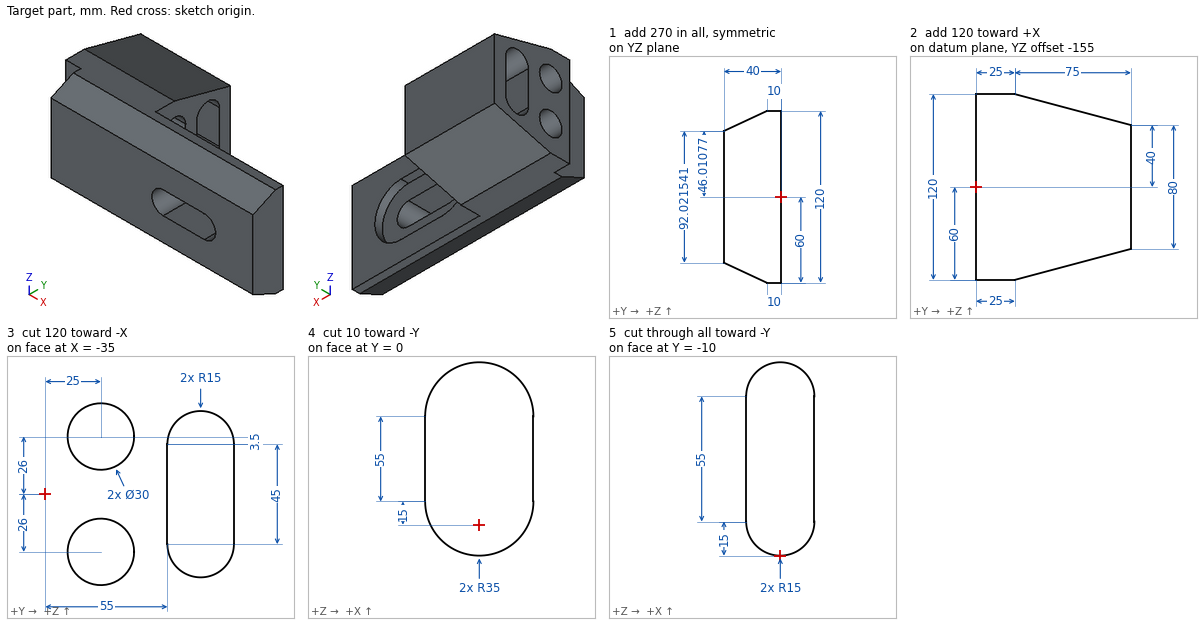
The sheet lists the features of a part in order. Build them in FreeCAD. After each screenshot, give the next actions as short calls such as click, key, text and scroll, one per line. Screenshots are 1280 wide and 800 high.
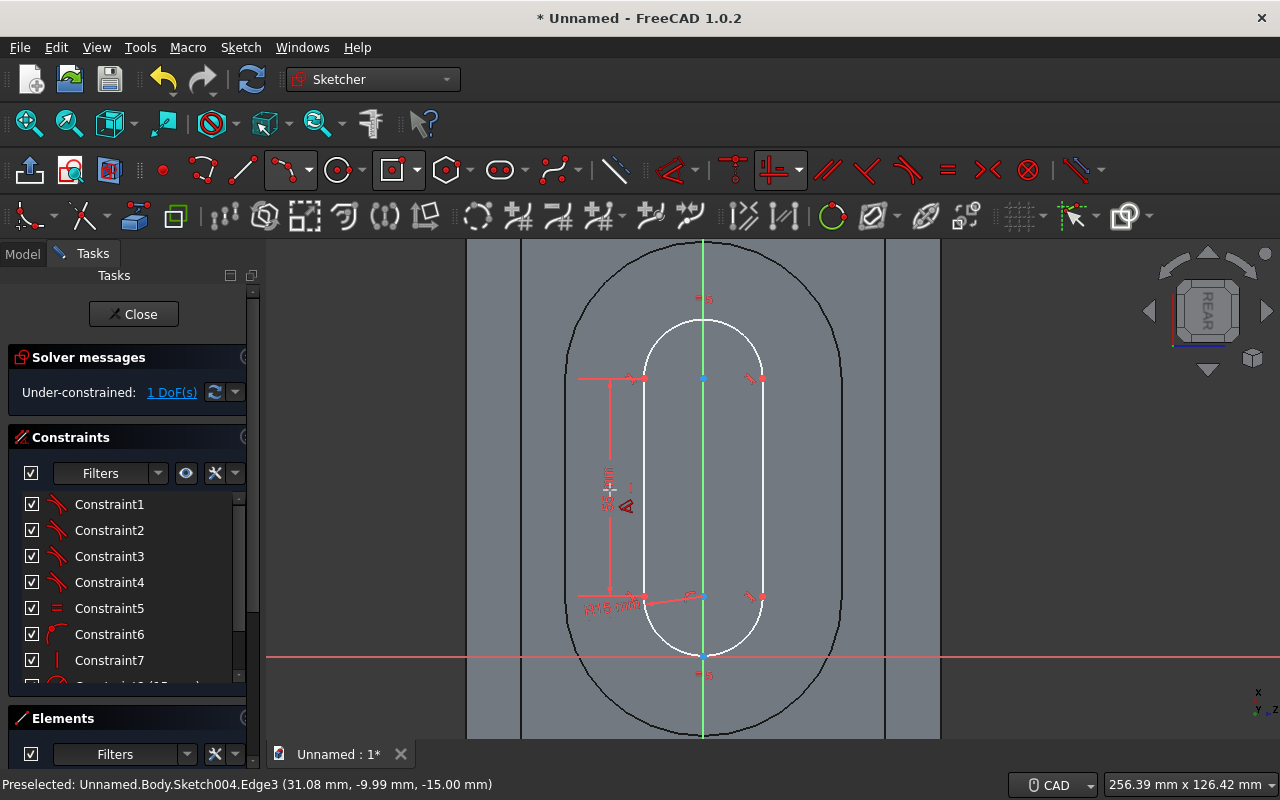
click(644, 596)
click(610, 641)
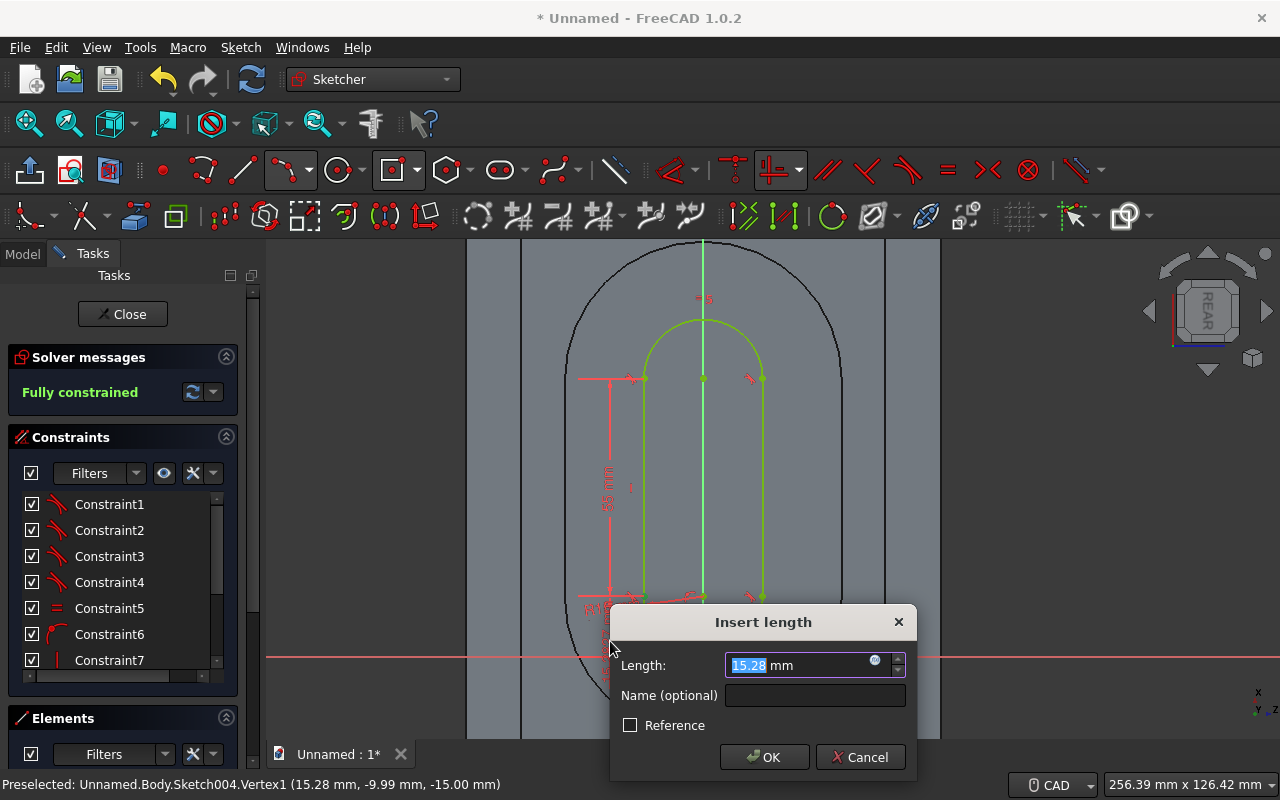
text(15)
key(Return)
key(Escape)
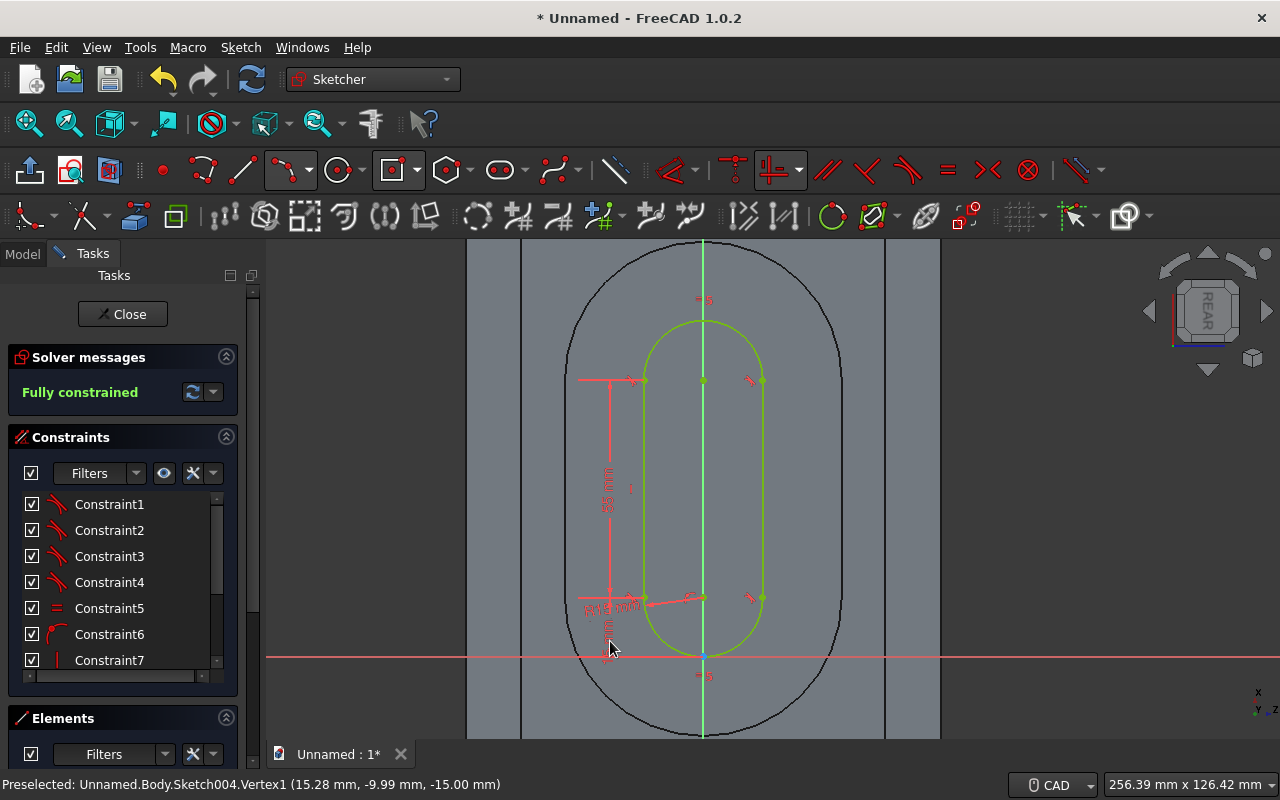
click(123, 314)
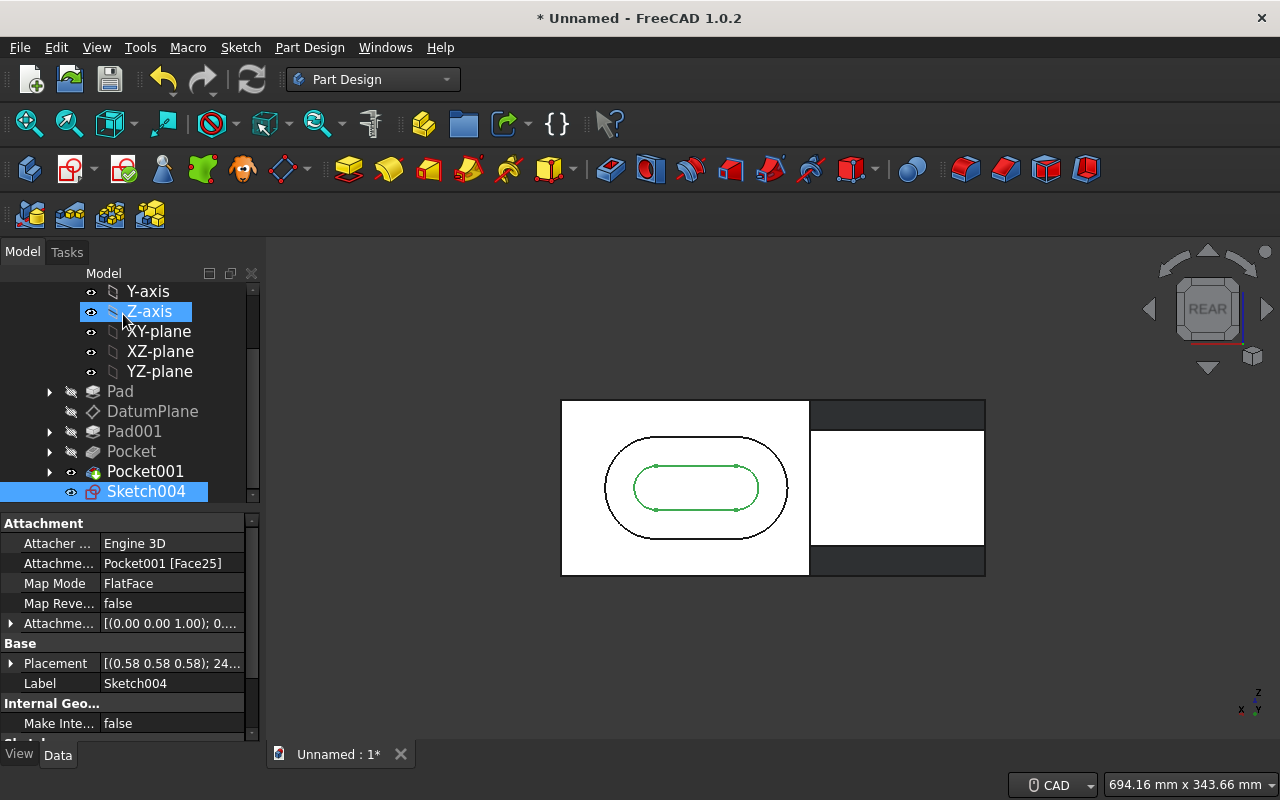
click(612, 170)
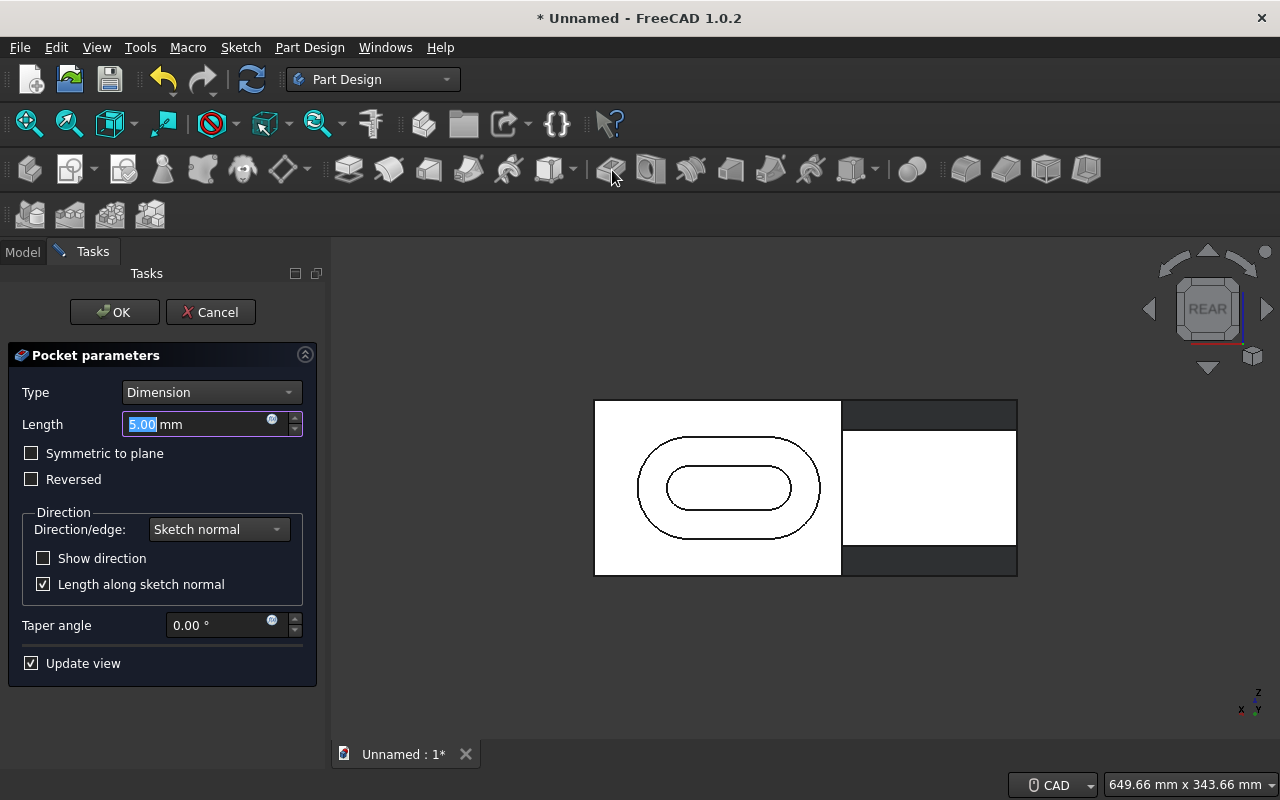
click(212, 392)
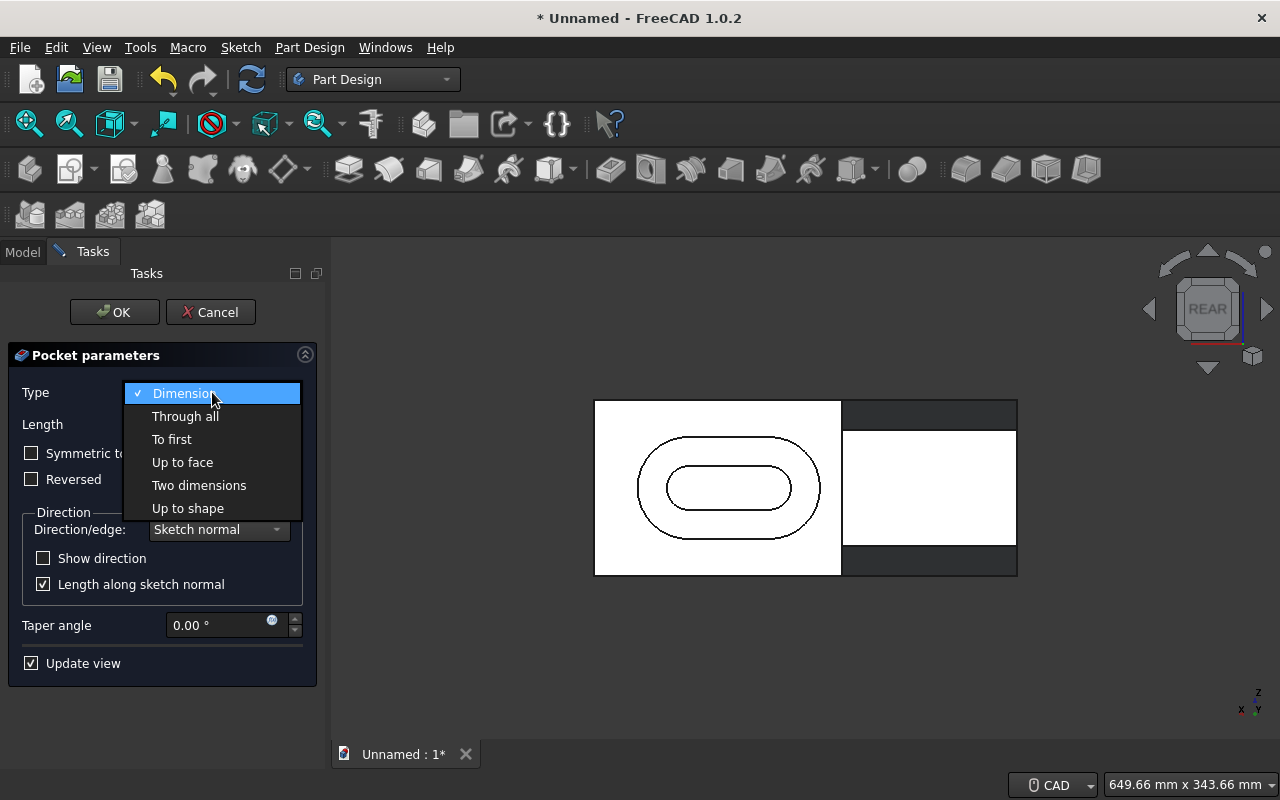
click(212, 416)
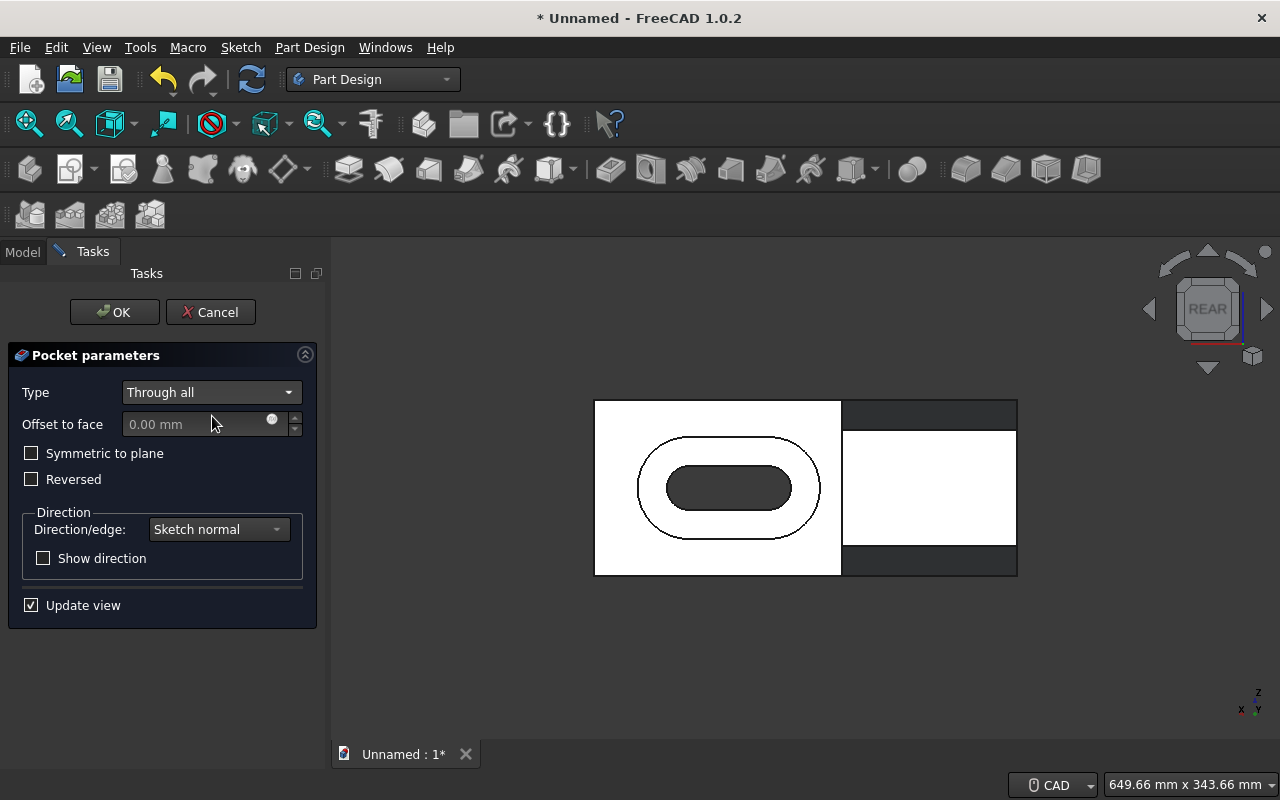
click(115, 312)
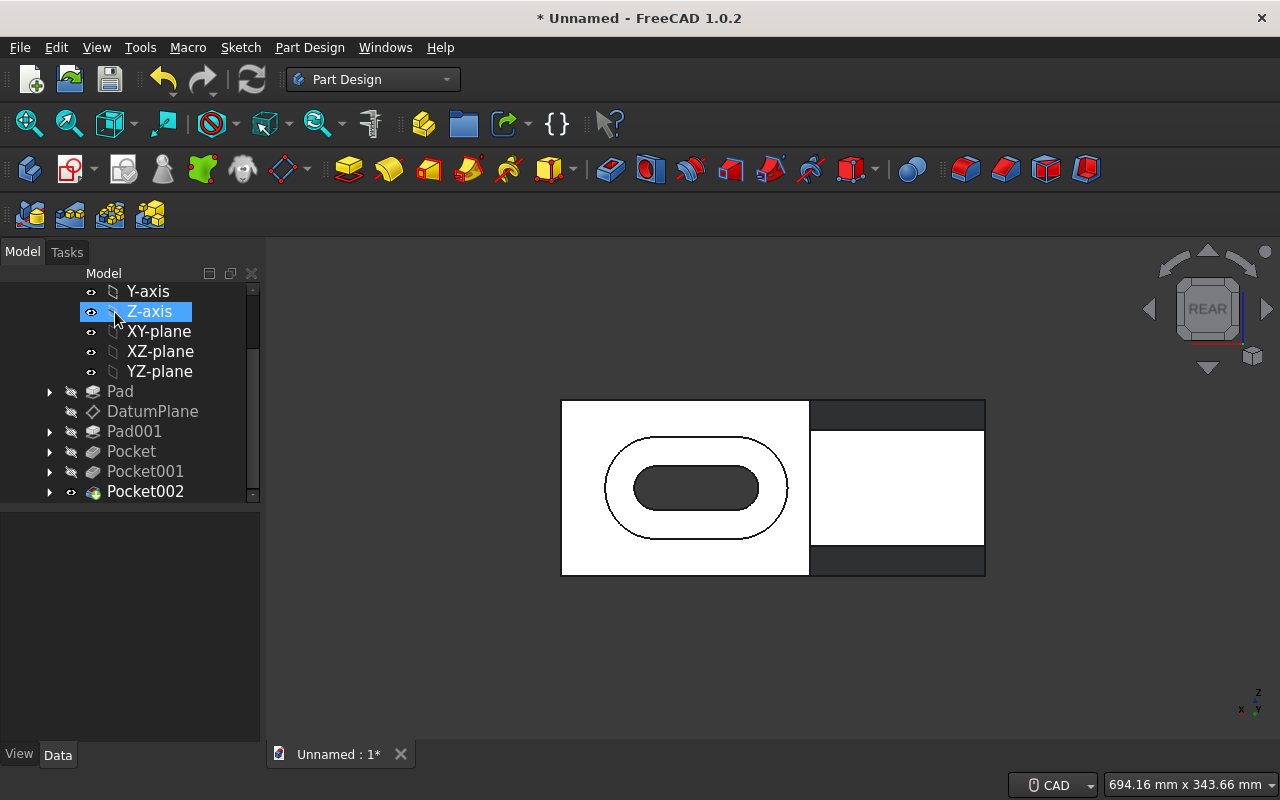
key(0)